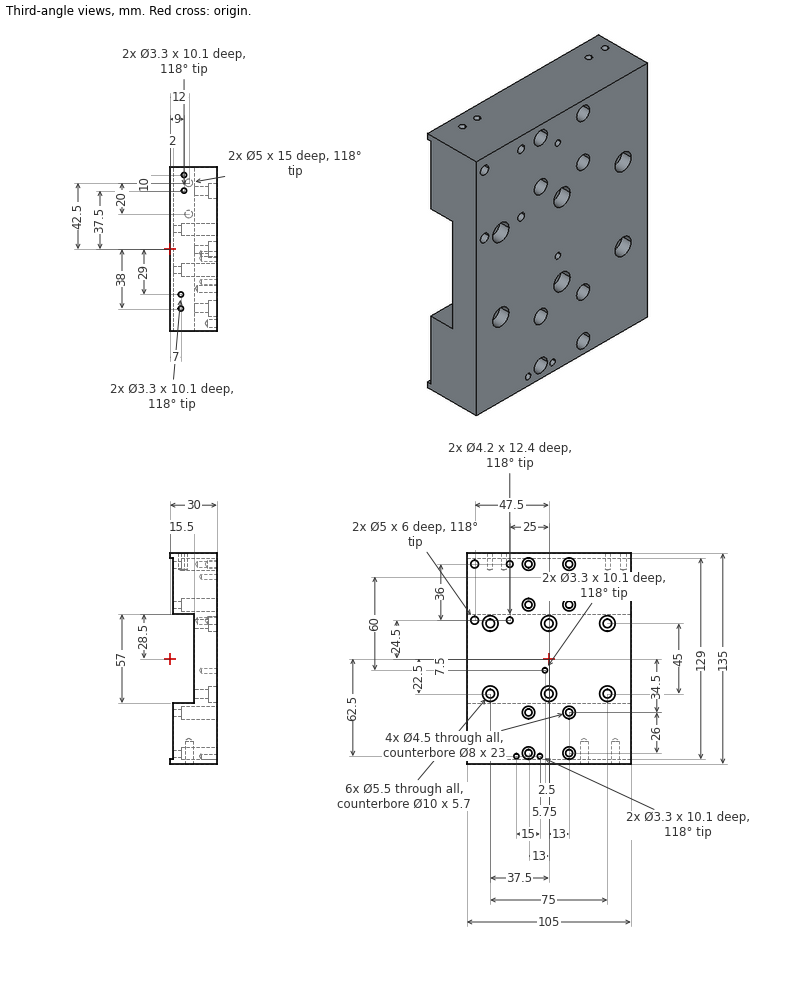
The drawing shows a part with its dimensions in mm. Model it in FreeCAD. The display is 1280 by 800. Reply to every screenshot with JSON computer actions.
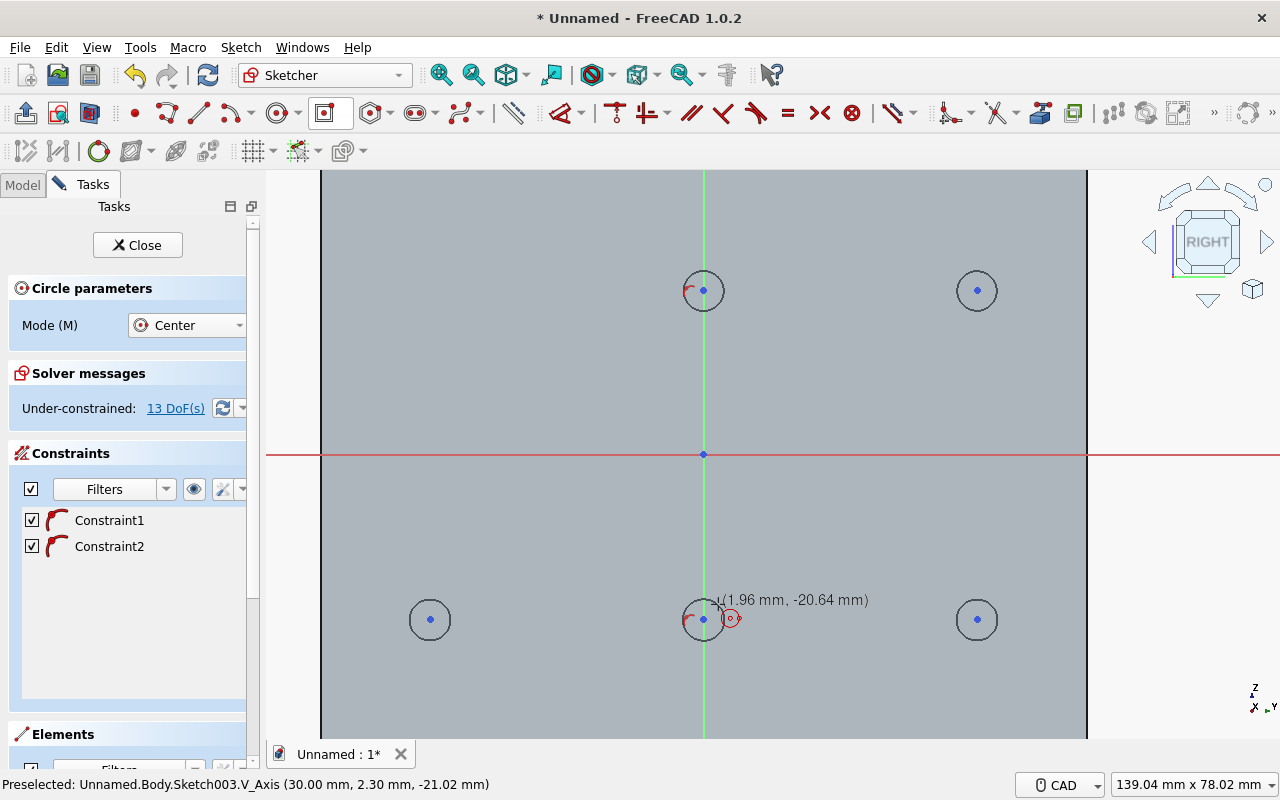
{"action": "left_click", "coordinate": [430, 290]}
{"action": "left_click", "coordinate": [444, 276]}
{"action": "key", "text": "Escape"}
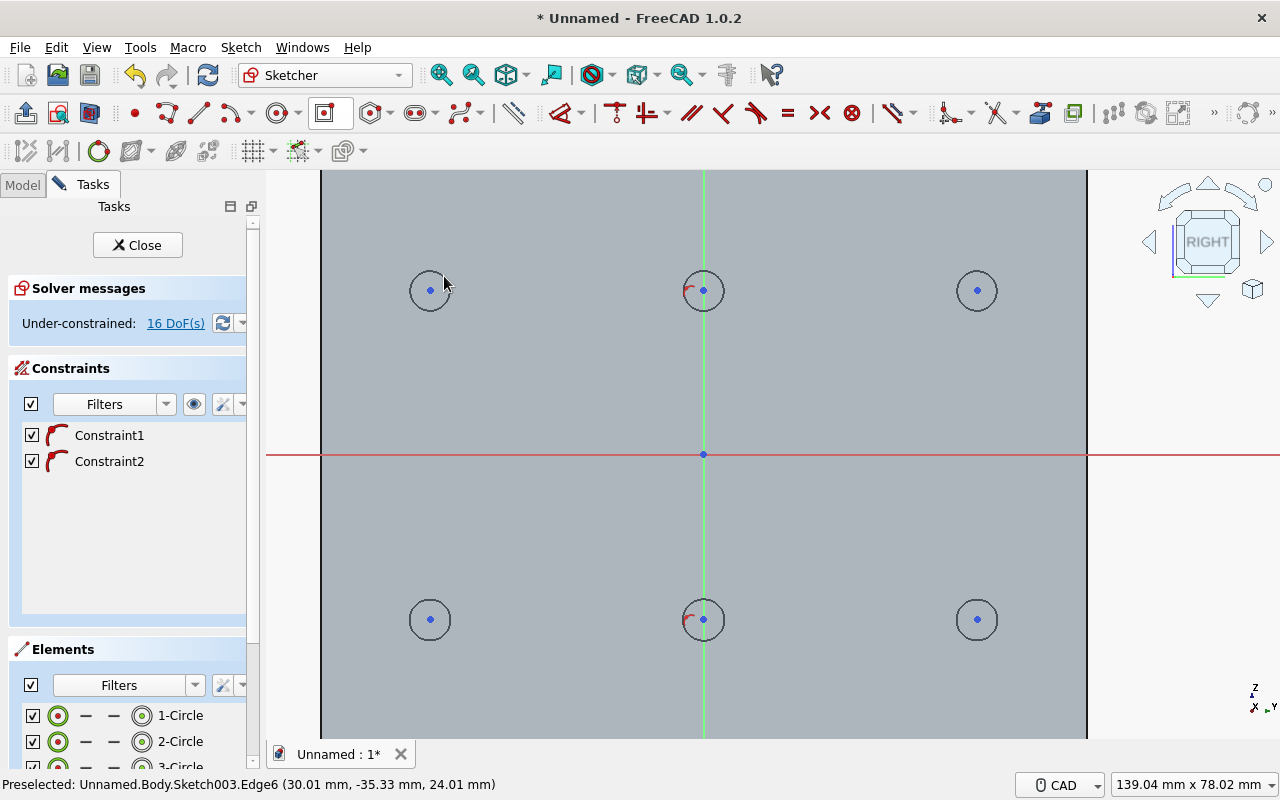
{"action": "left_click", "coordinate": [444, 605]}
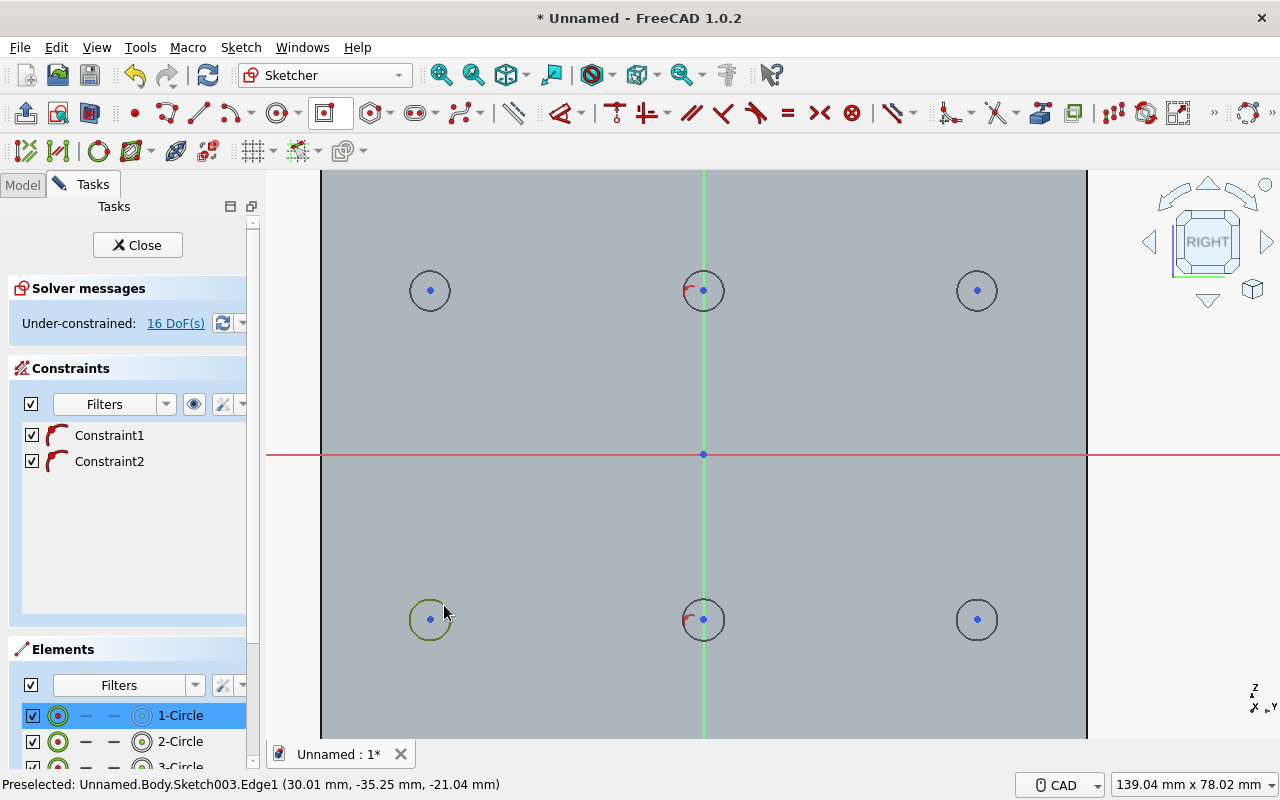
{"action": "left_click", "coordinate": [991, 605]}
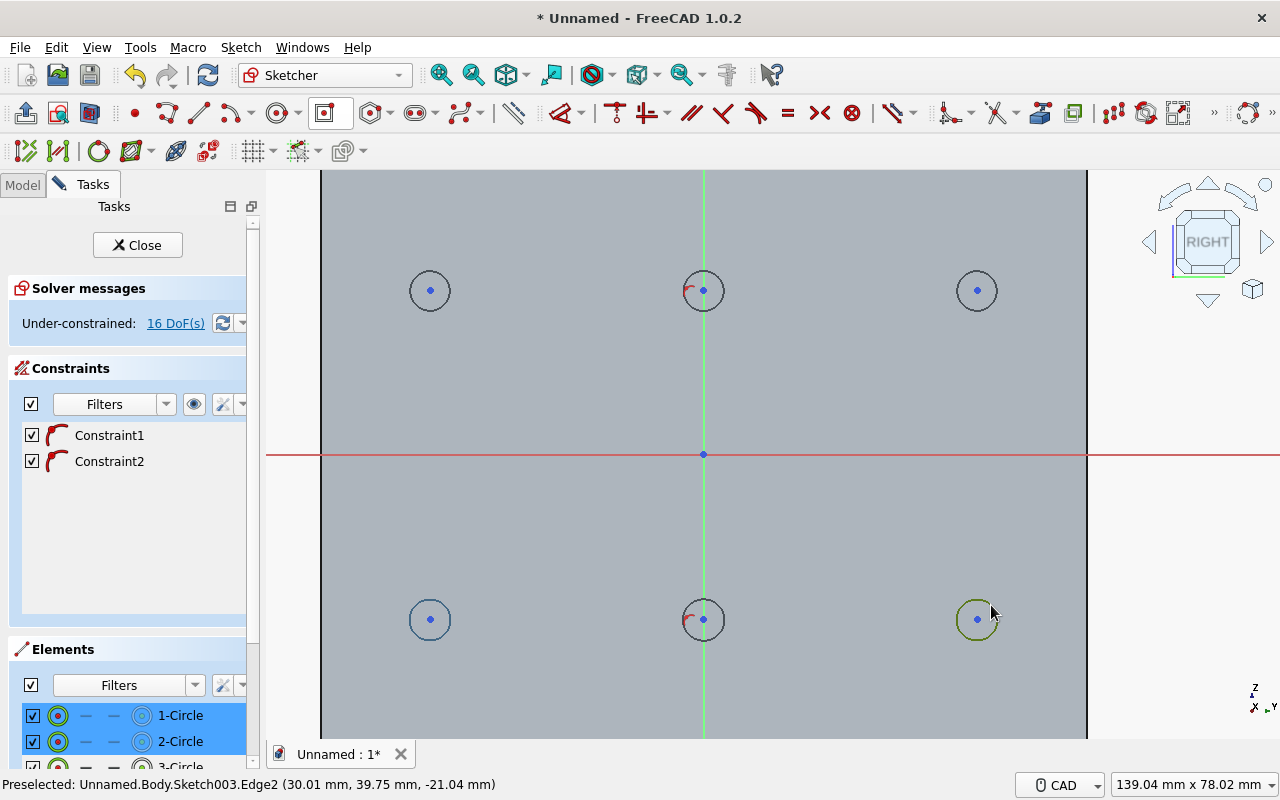
{"action": "left_click", "coordinate": [991, 277]}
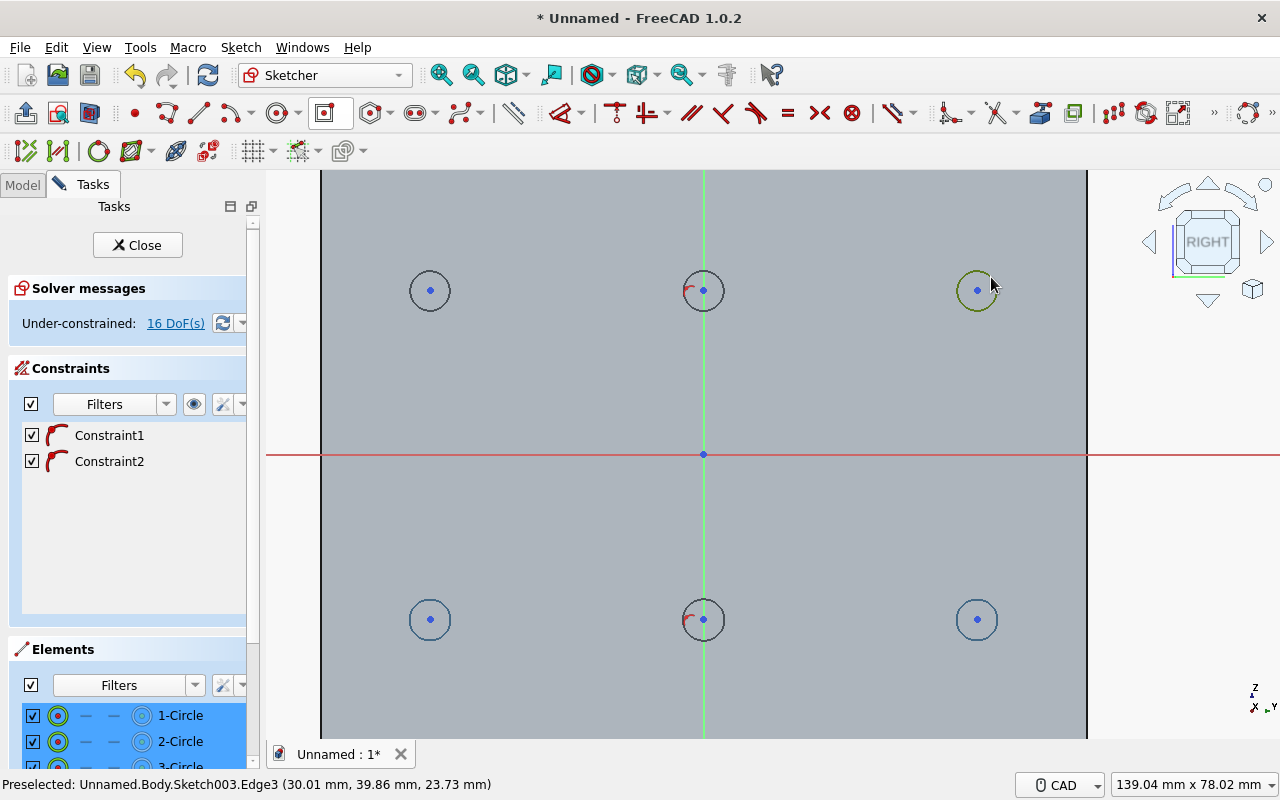
{"action": "left_click", "coordinate": [718, 277]}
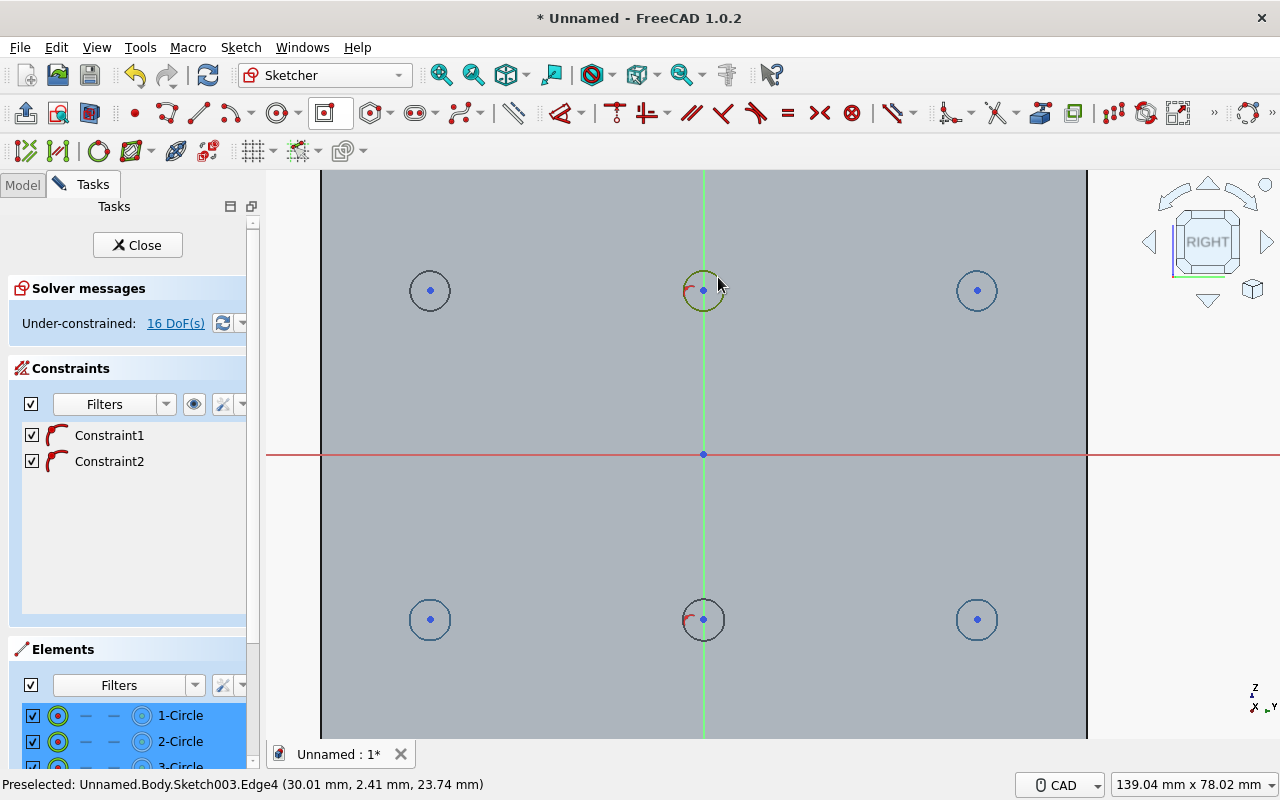
{"action": "left_click", "coordinate": [718, 605]}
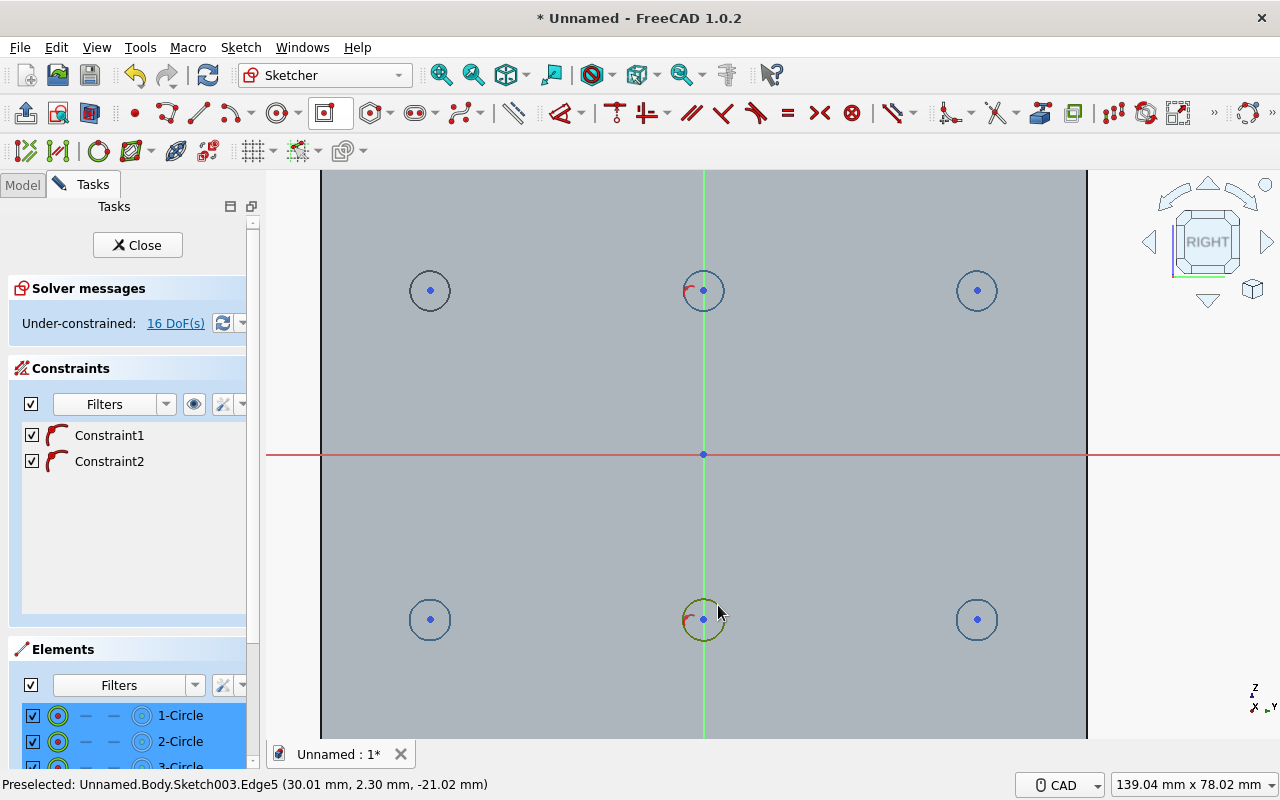
{"action": "left_click", "coordinate": [444, 277]}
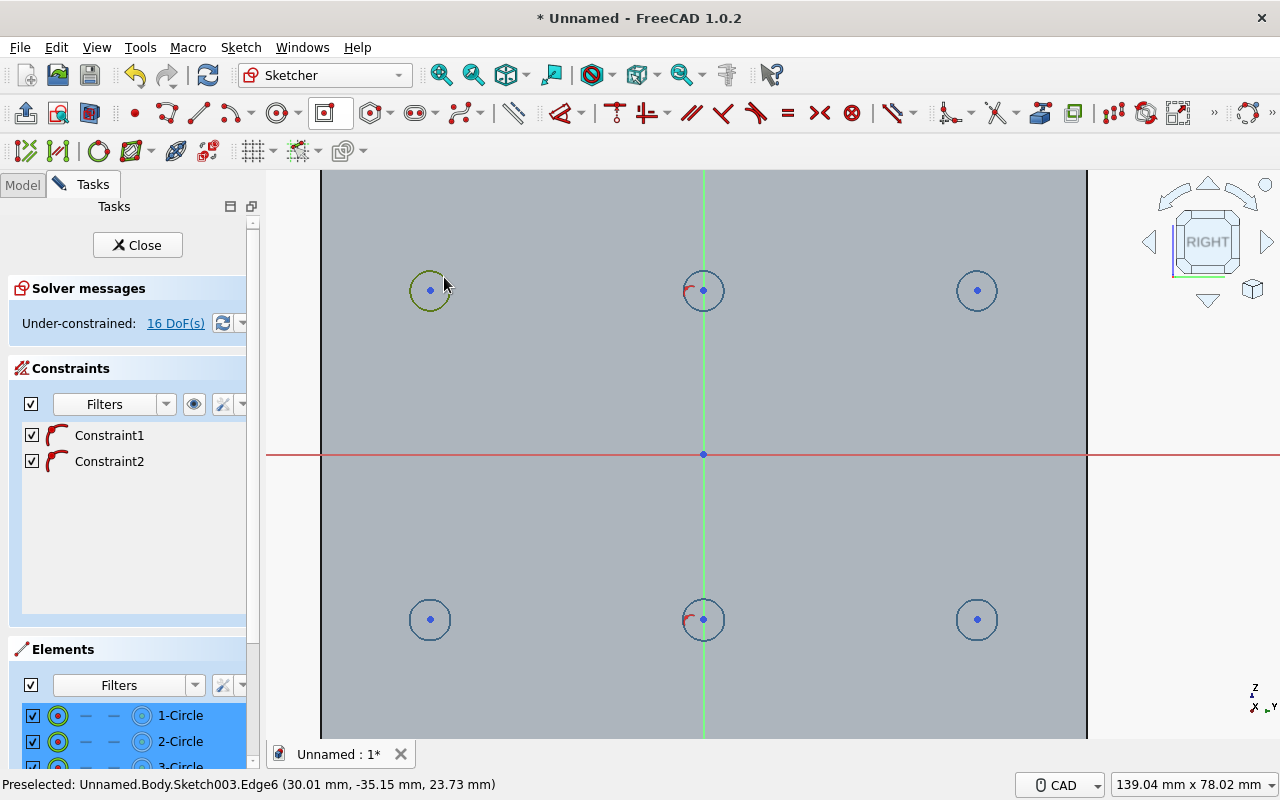
{"action": "left_click", "coordinate": [788, 114]}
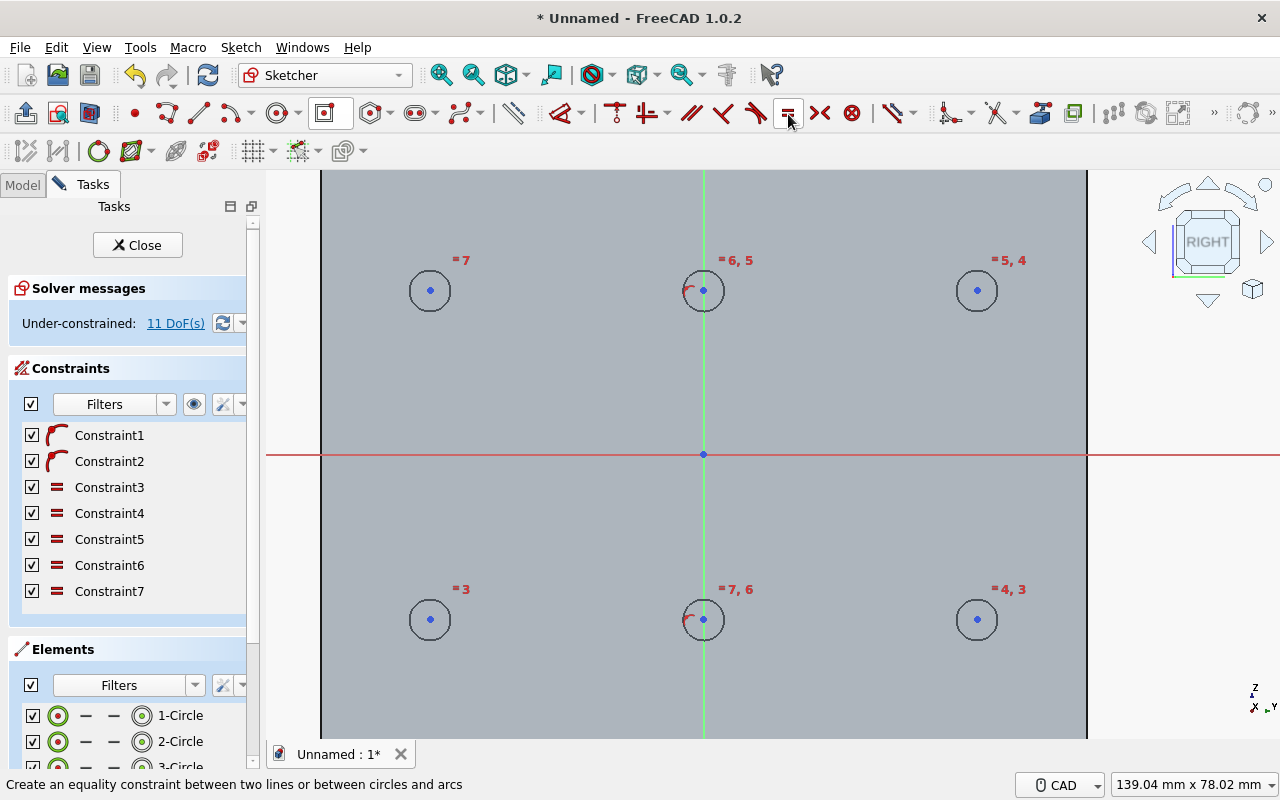
{"action": "left_click", "coordinate": [430, 620]}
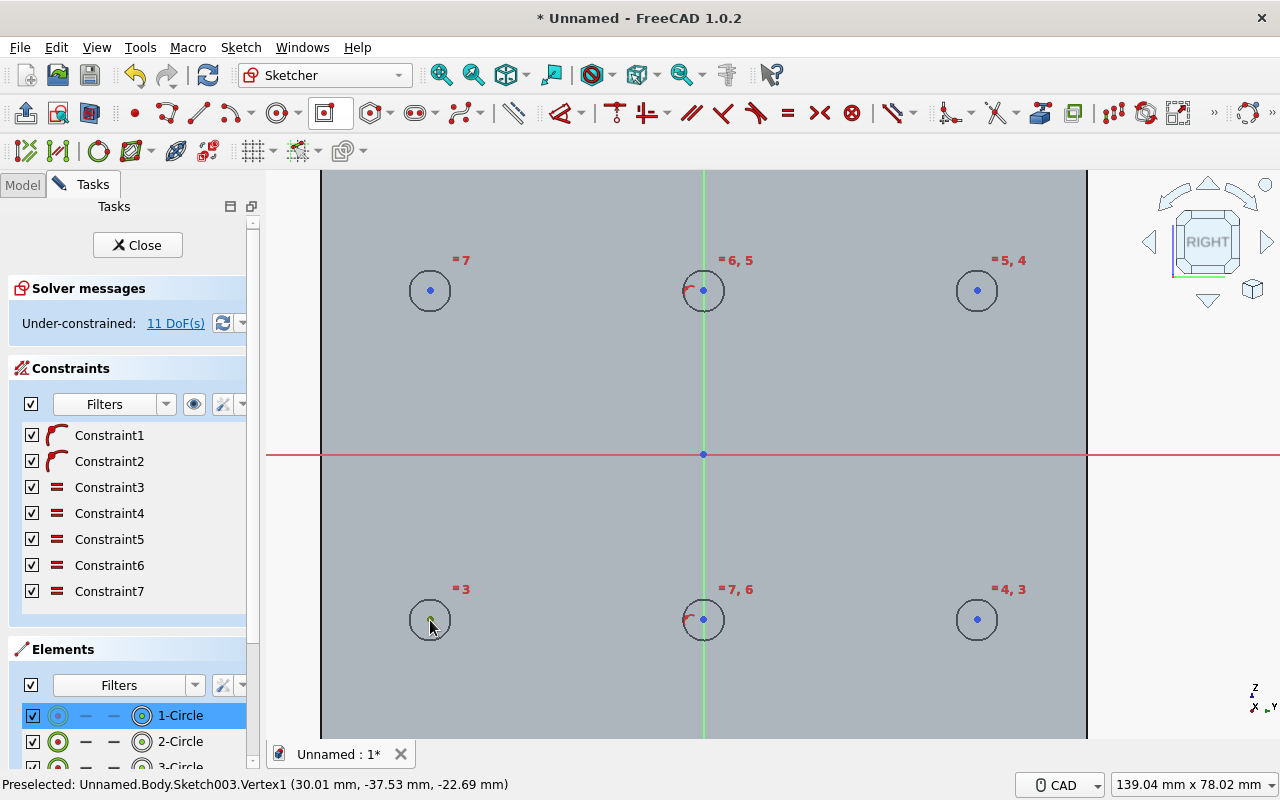
{"action": "left_click", "coordinate": [977, 620]}